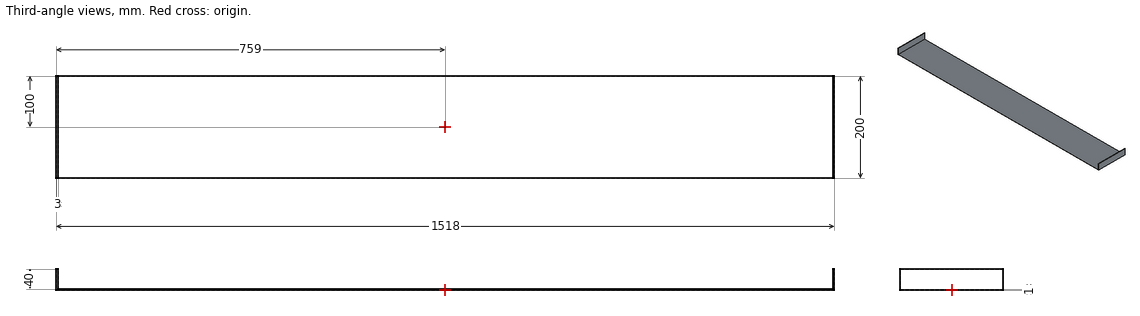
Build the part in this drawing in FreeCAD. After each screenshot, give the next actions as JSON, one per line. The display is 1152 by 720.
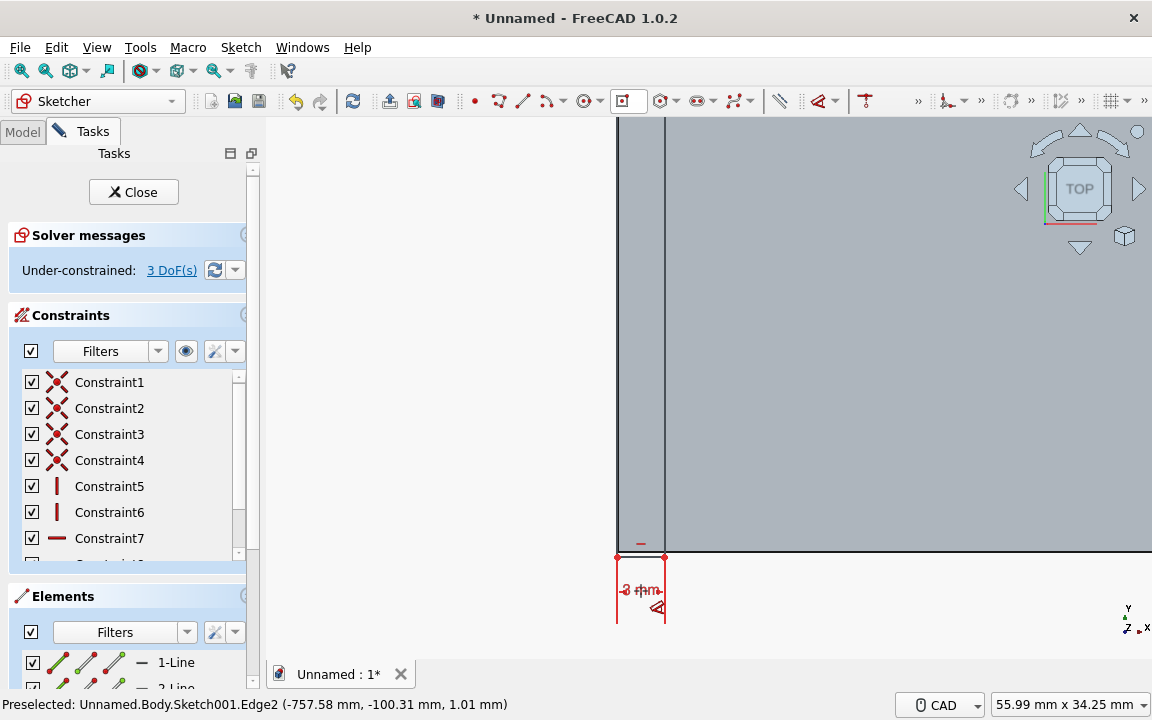
{"action": "scroll", "coordinate": [640, 565], "scroll_direction": "down", "scroll_amount": 11}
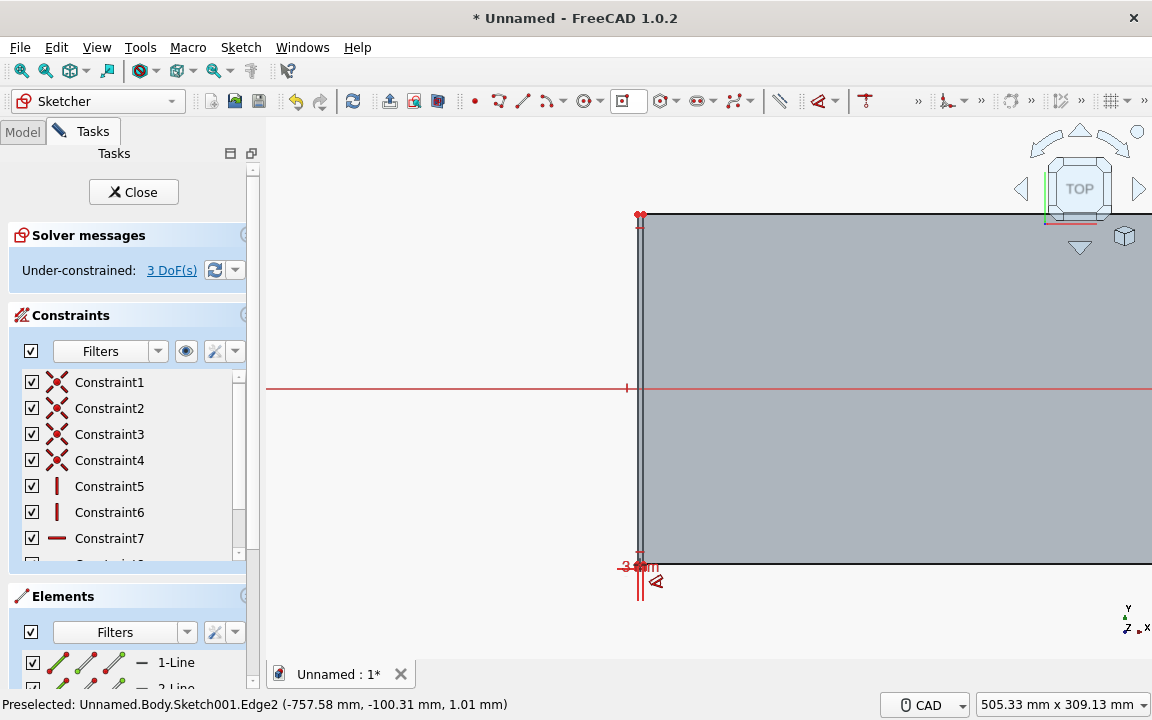
{"action": "scroll", "coordinate": [638, 319], "scroll_direction": "up", "scroll_amount": 5}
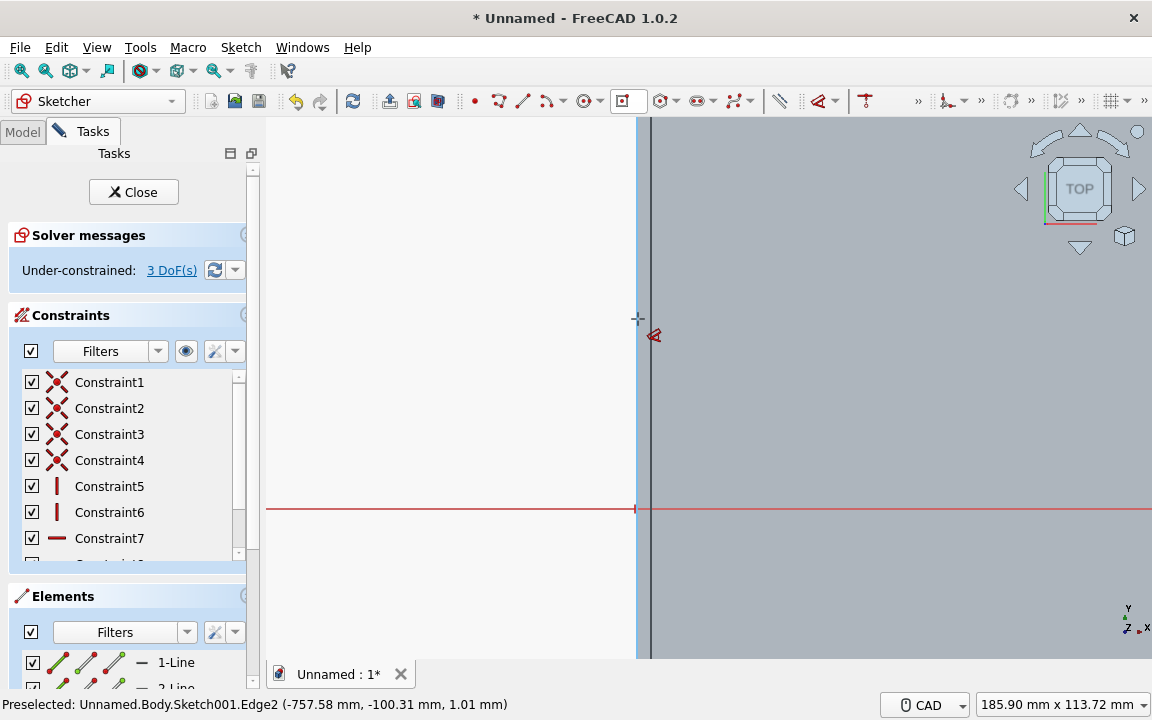
{"action": "left_click", "coordinate": [637, 319]}
{"action": "left_click", "coordinate": [603, 388]}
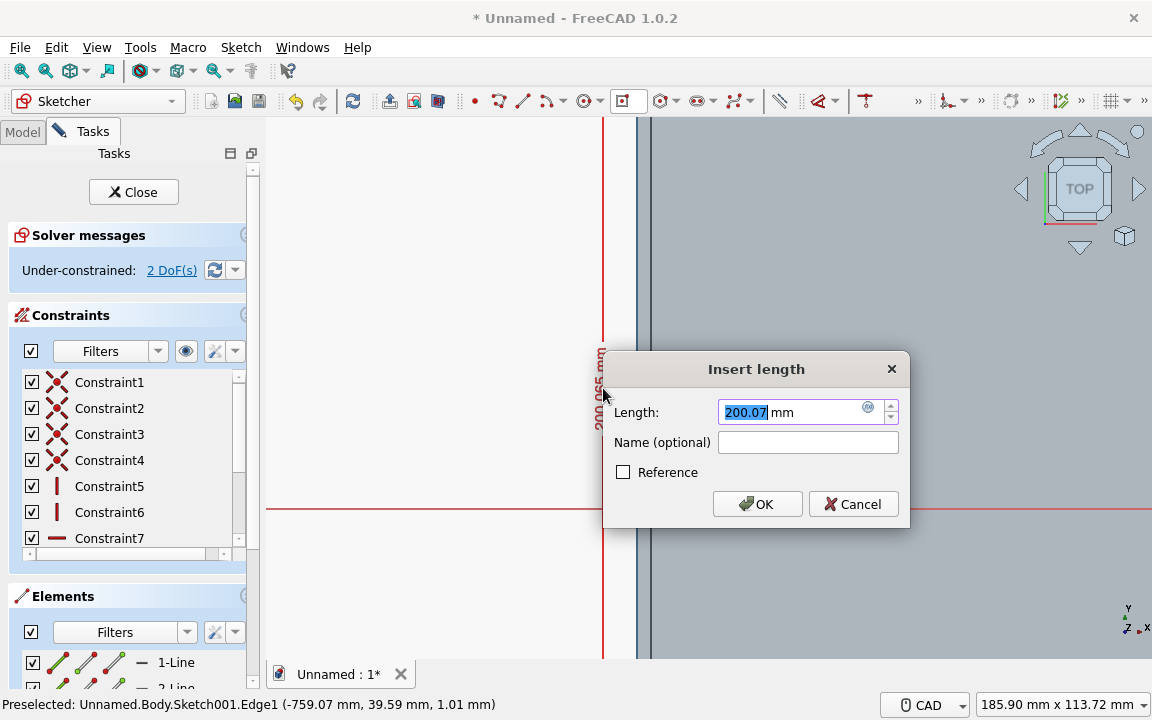
{"action": "type", "text": "200"}
{"action": "key", "text": "Return"}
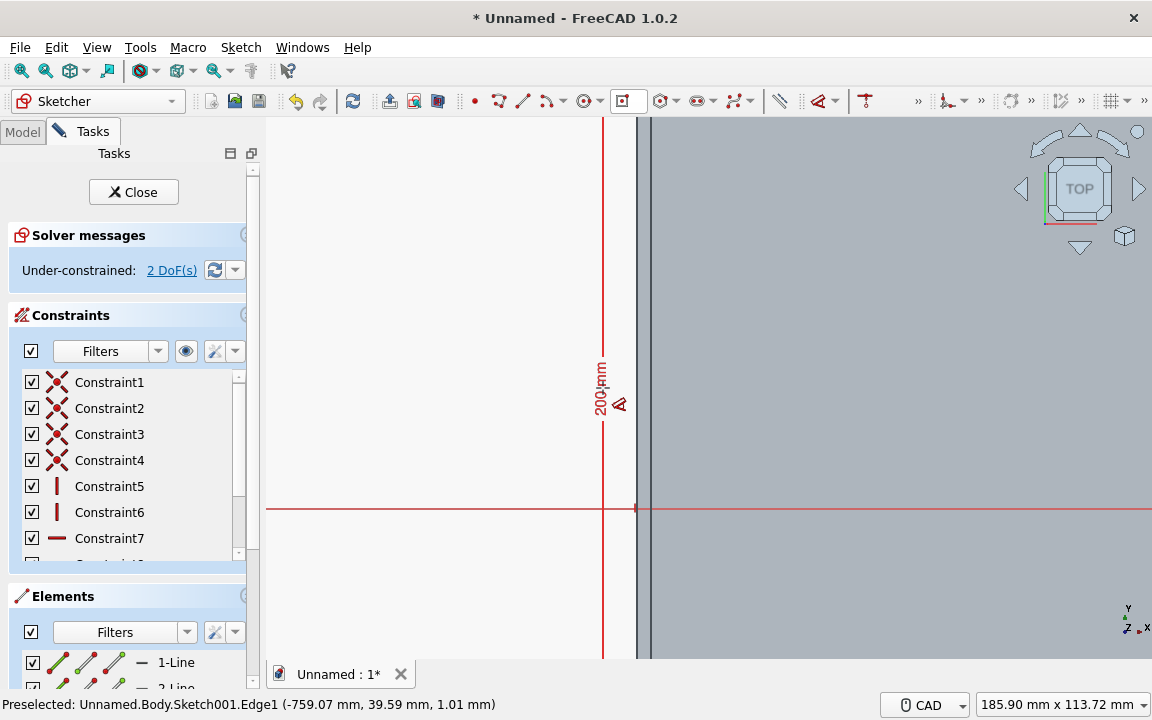
{"action": "scroll", "coordinate": [638, 318], "scroll_direction": "down", "scroll_amount": 5}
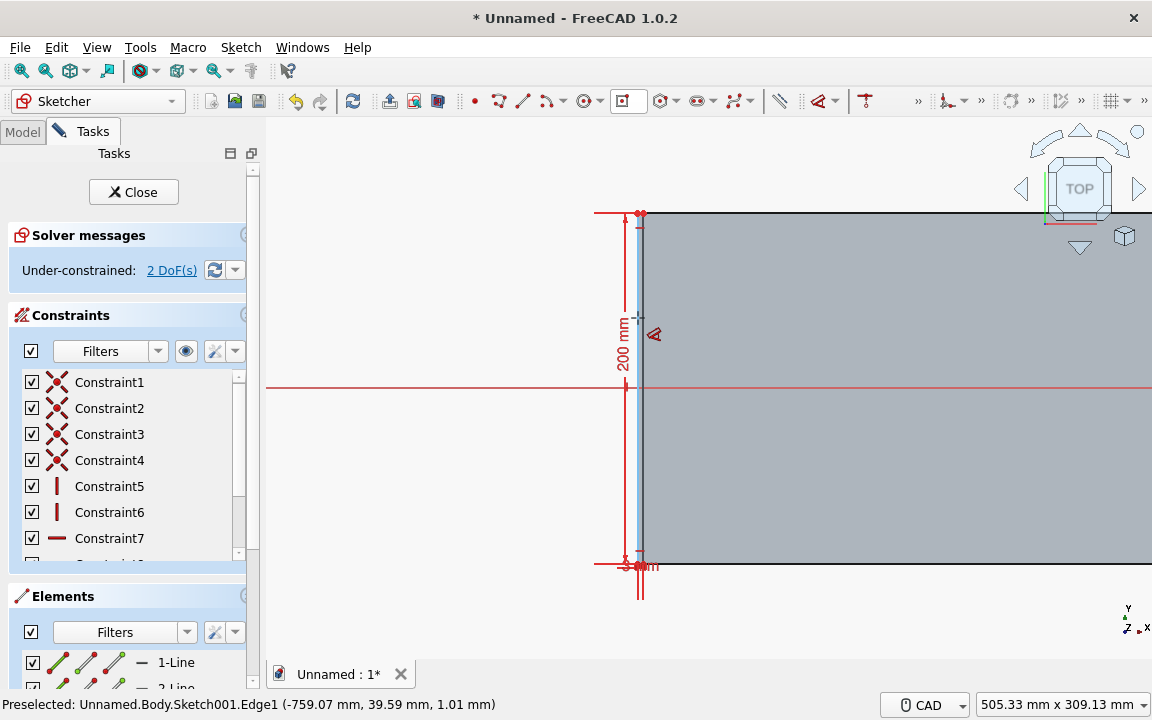
{"action": "scroll", "coordinate": [638, 213], "scroll_direction": "up", "scroll_amount": 5}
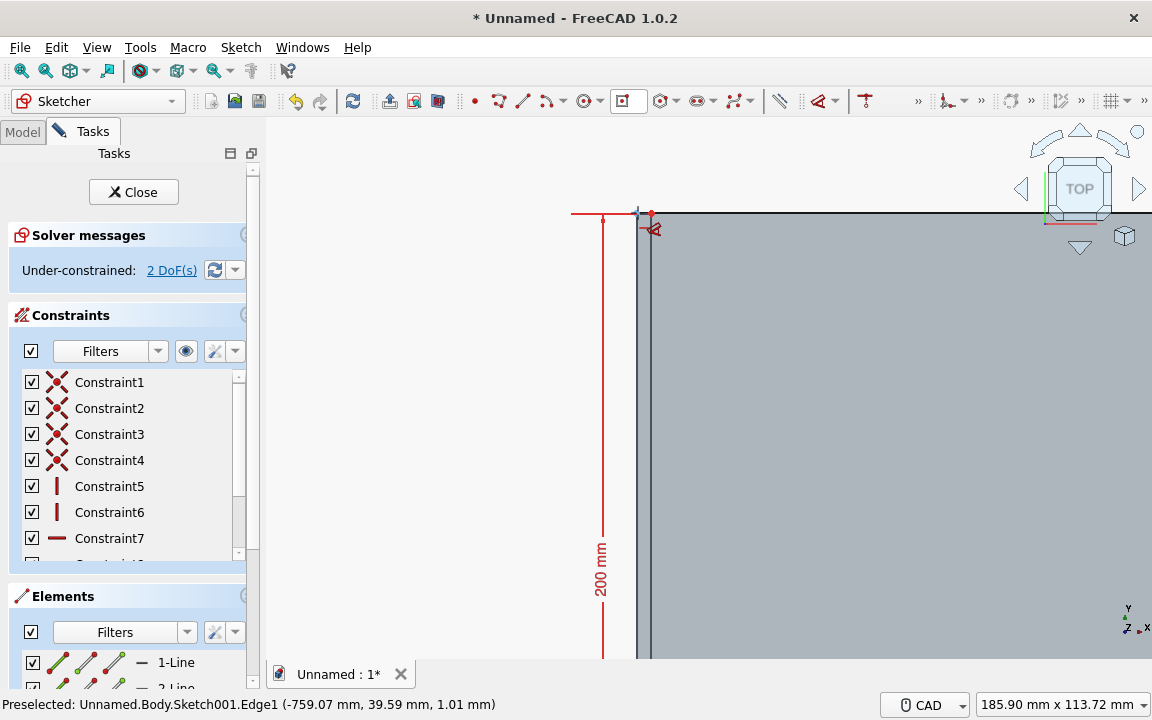
{"action": "left_click", "coordinate": [637, 214]}
{"action": "left_click", "coordinate": [812, 180]}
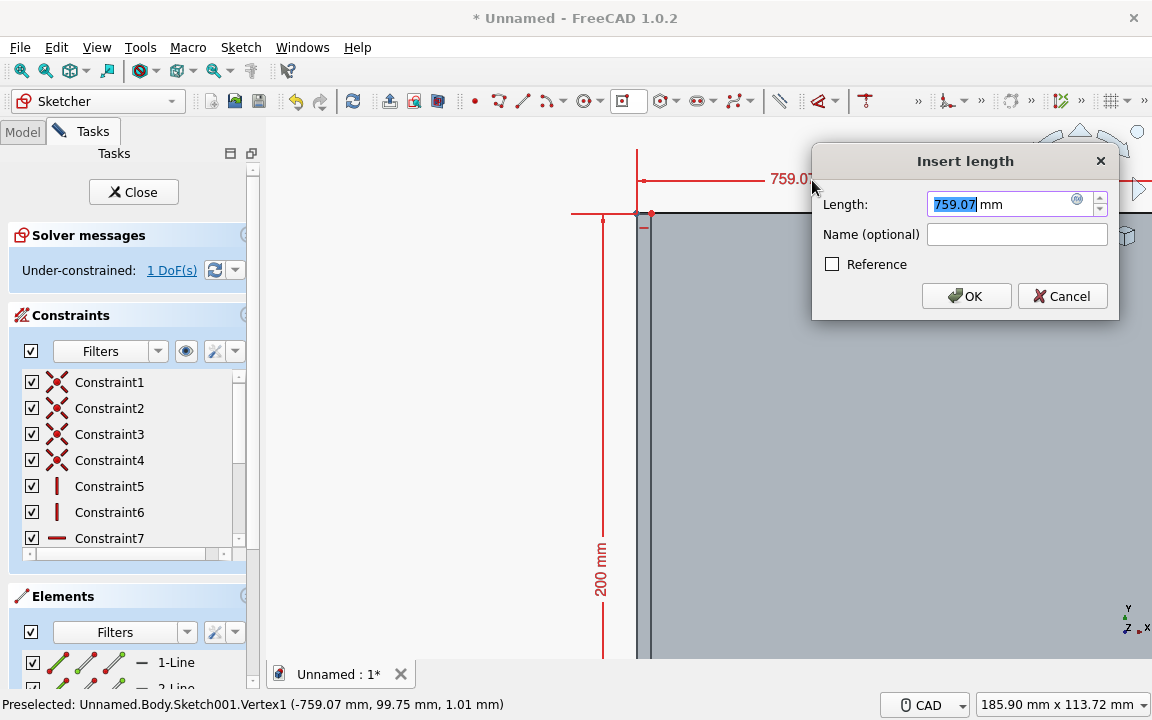
{"action": "type", "text": "759"}
{"action": "key", "text": "Return"}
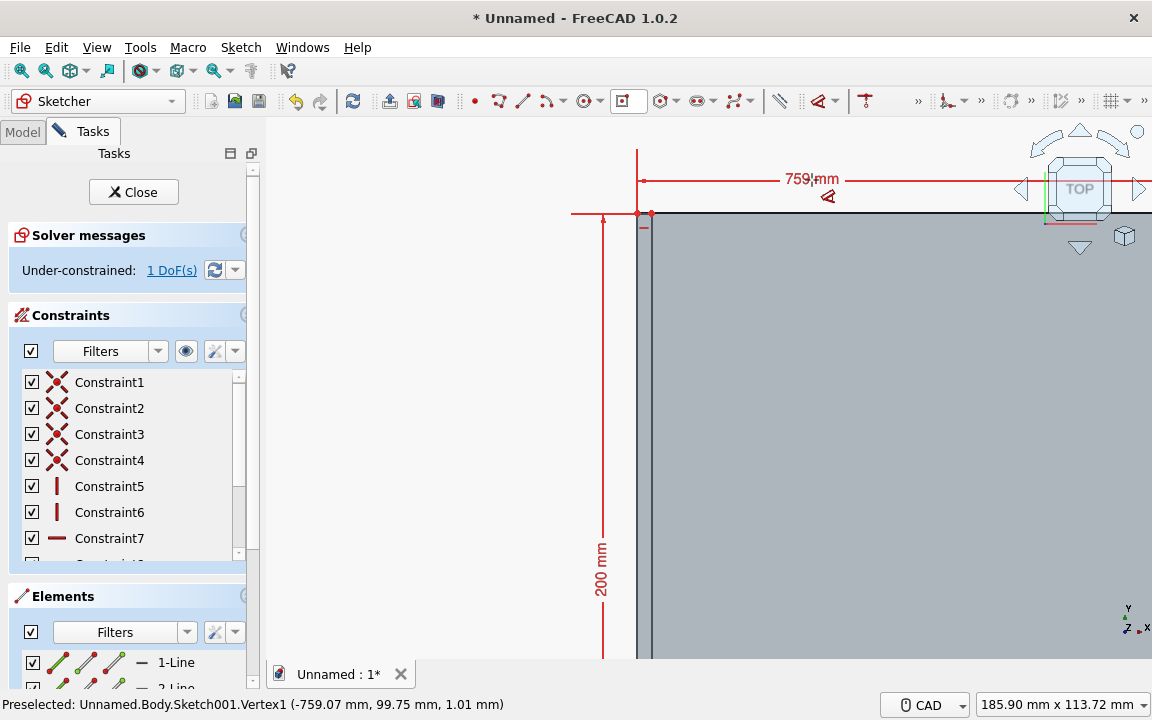
{"action": "left_click", "coordinate": [637, 214]}
{"action": "left_click", "coordinate": [603, 422]}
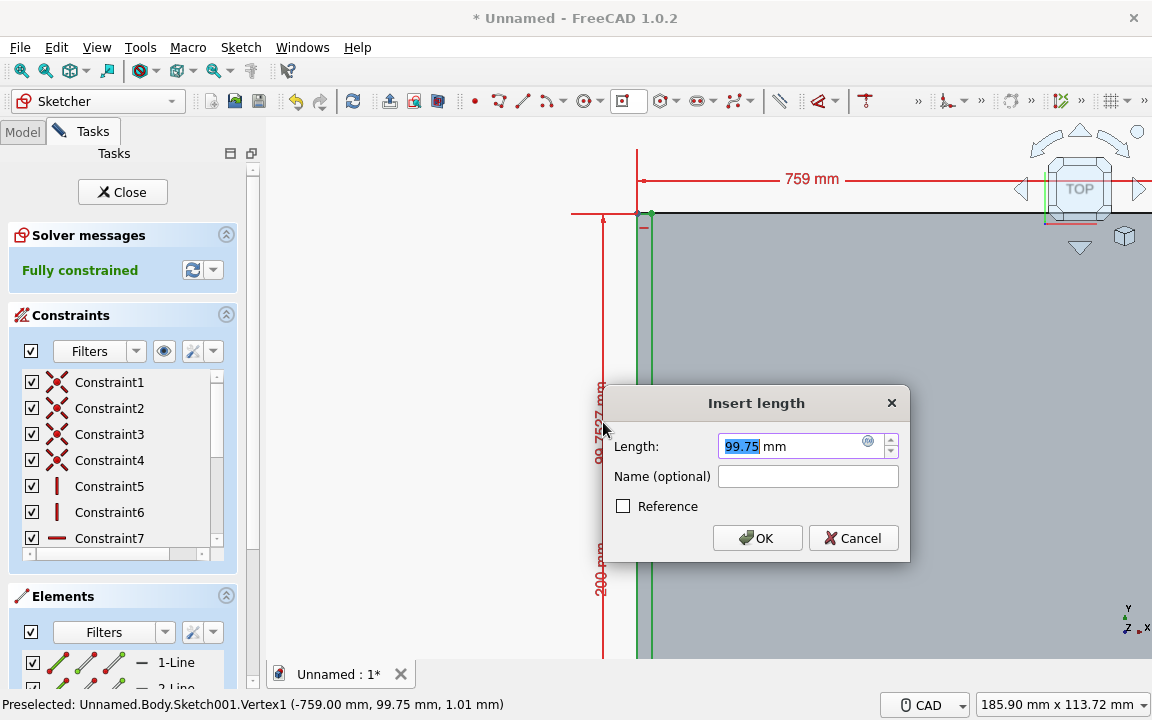
{"action": "type", "text": "100"}
{"action": "key", "text": "Return"}
{"action": "key", "text": "Escape"}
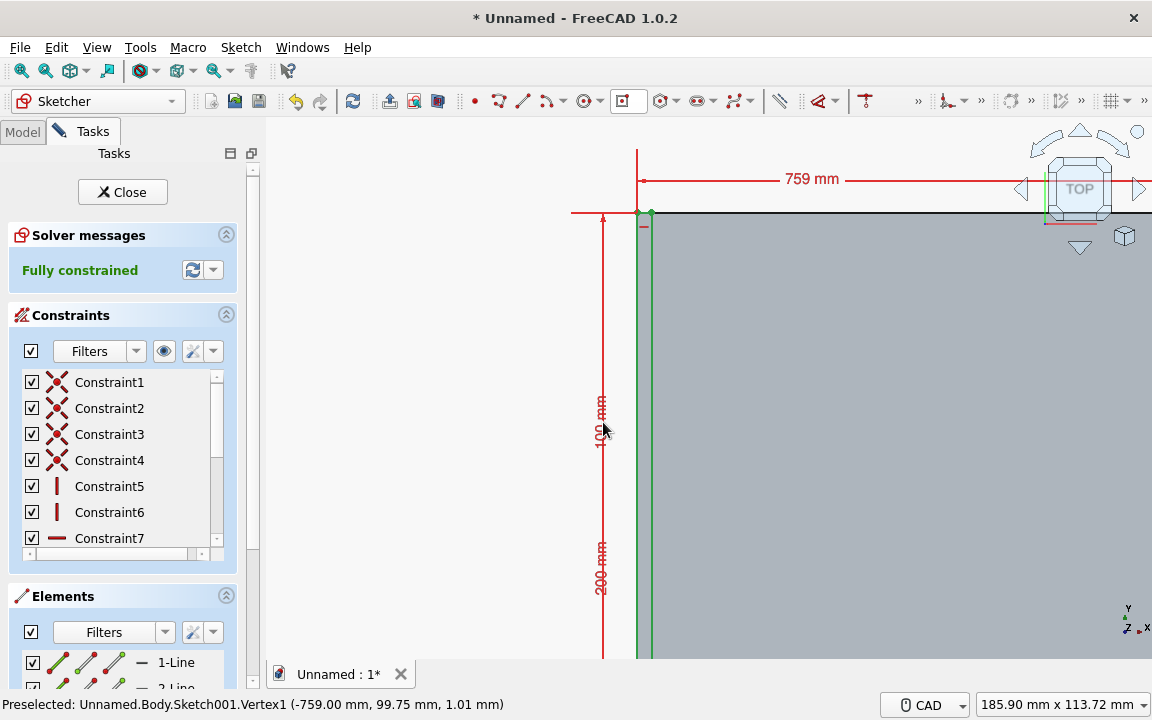
{"action": "left_click", "coordinate": [123, 192]}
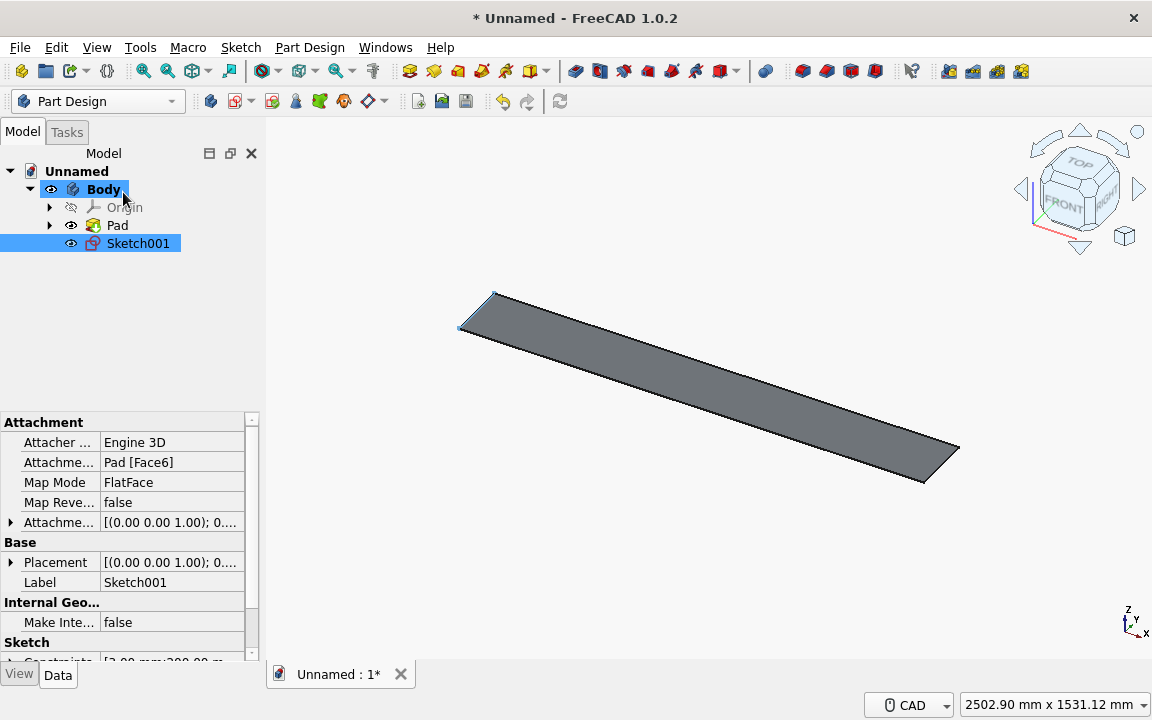
{"action": "left_click", "coordinate": [410, 72]}